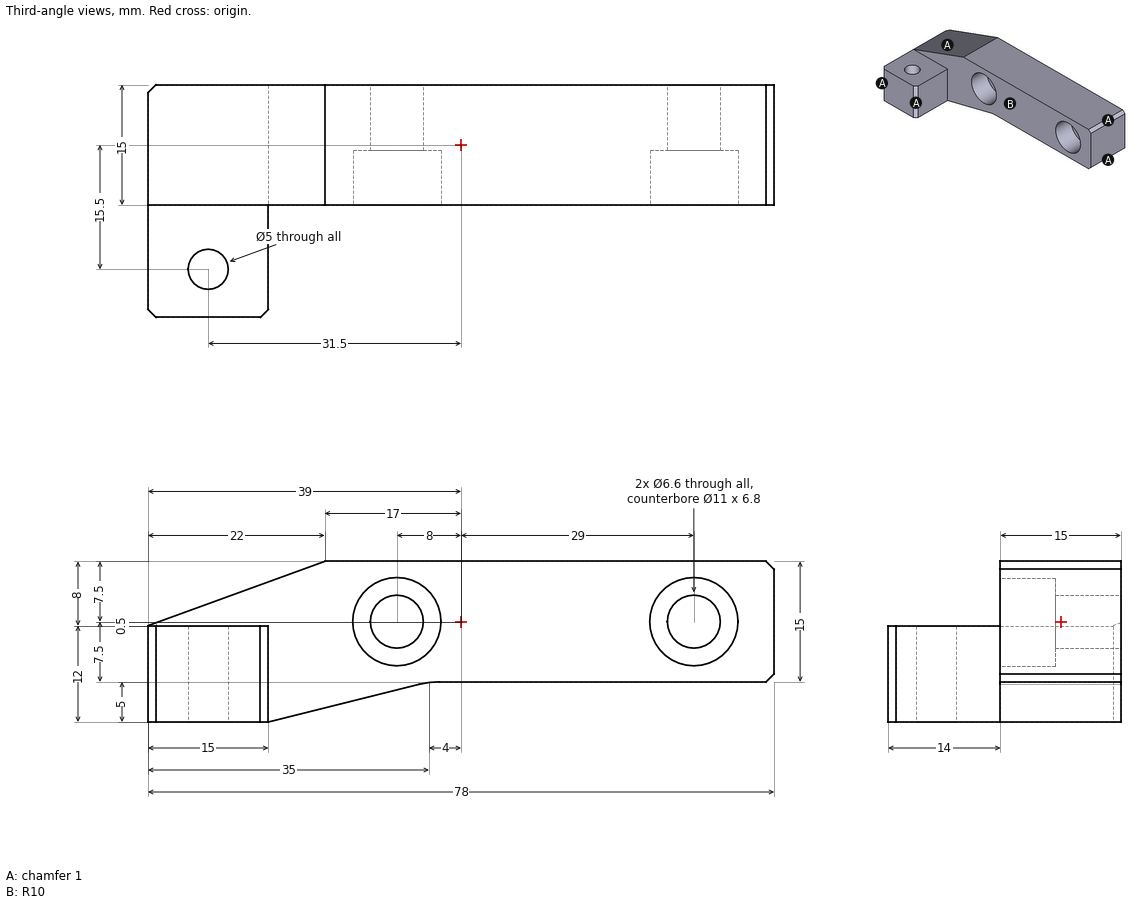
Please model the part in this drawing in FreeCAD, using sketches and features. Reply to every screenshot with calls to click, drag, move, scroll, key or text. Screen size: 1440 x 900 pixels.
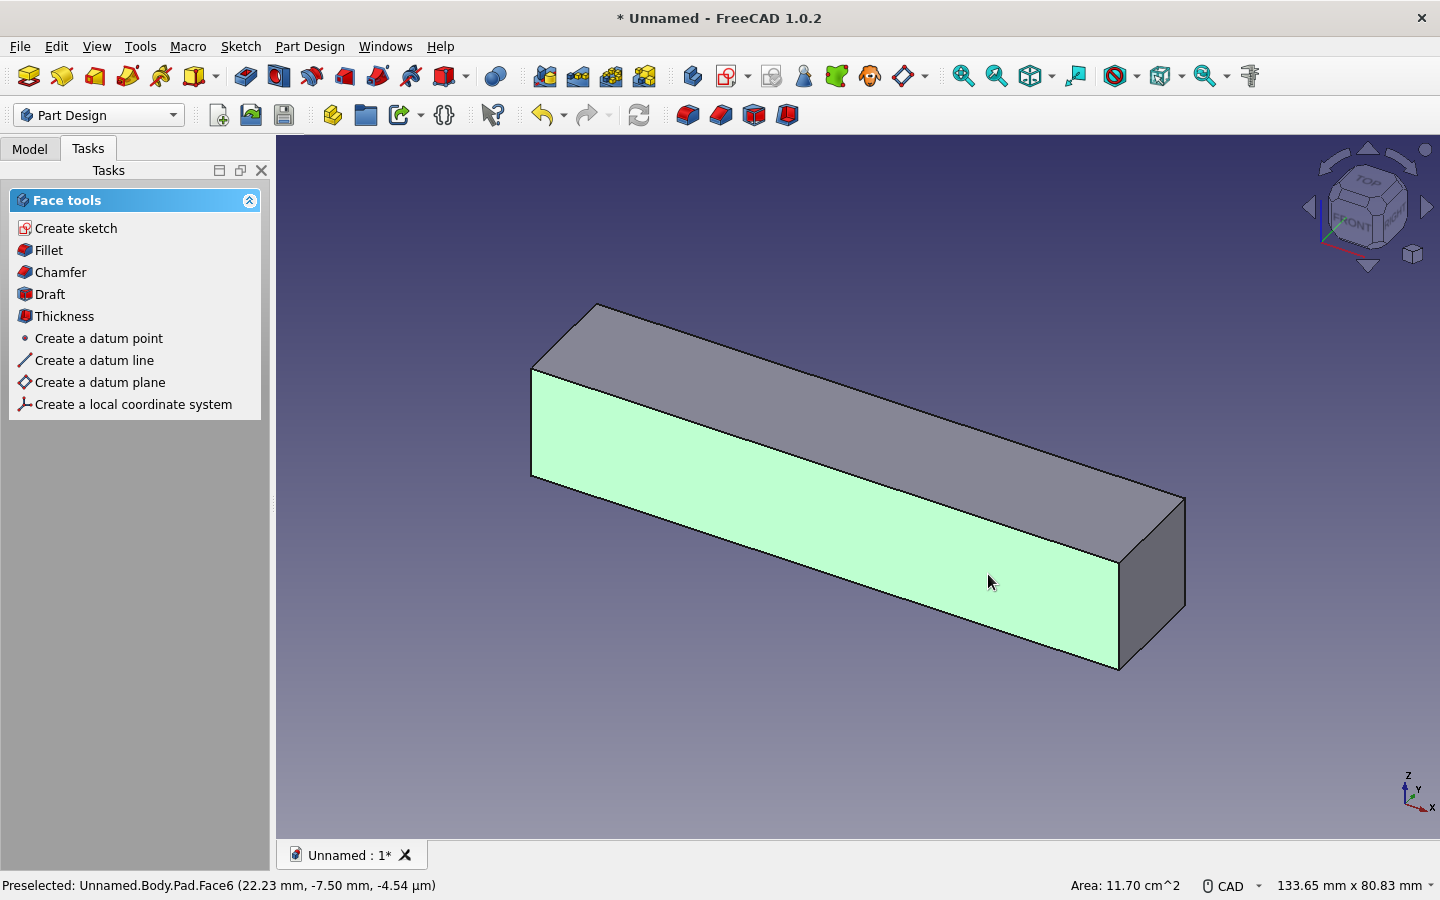
click(726, 76)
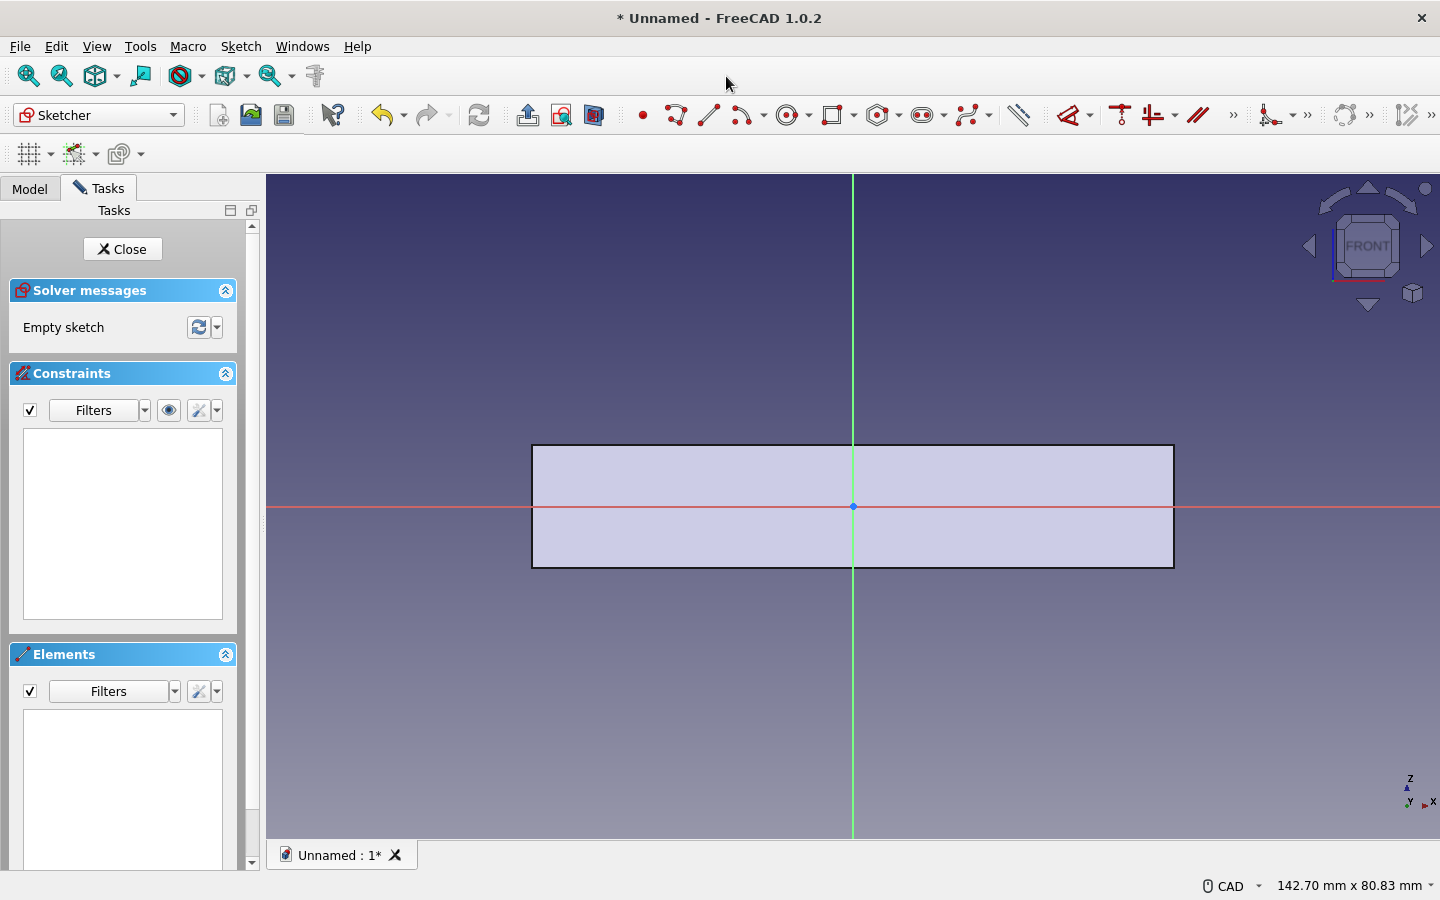
scroll(1128, 507, up, 3)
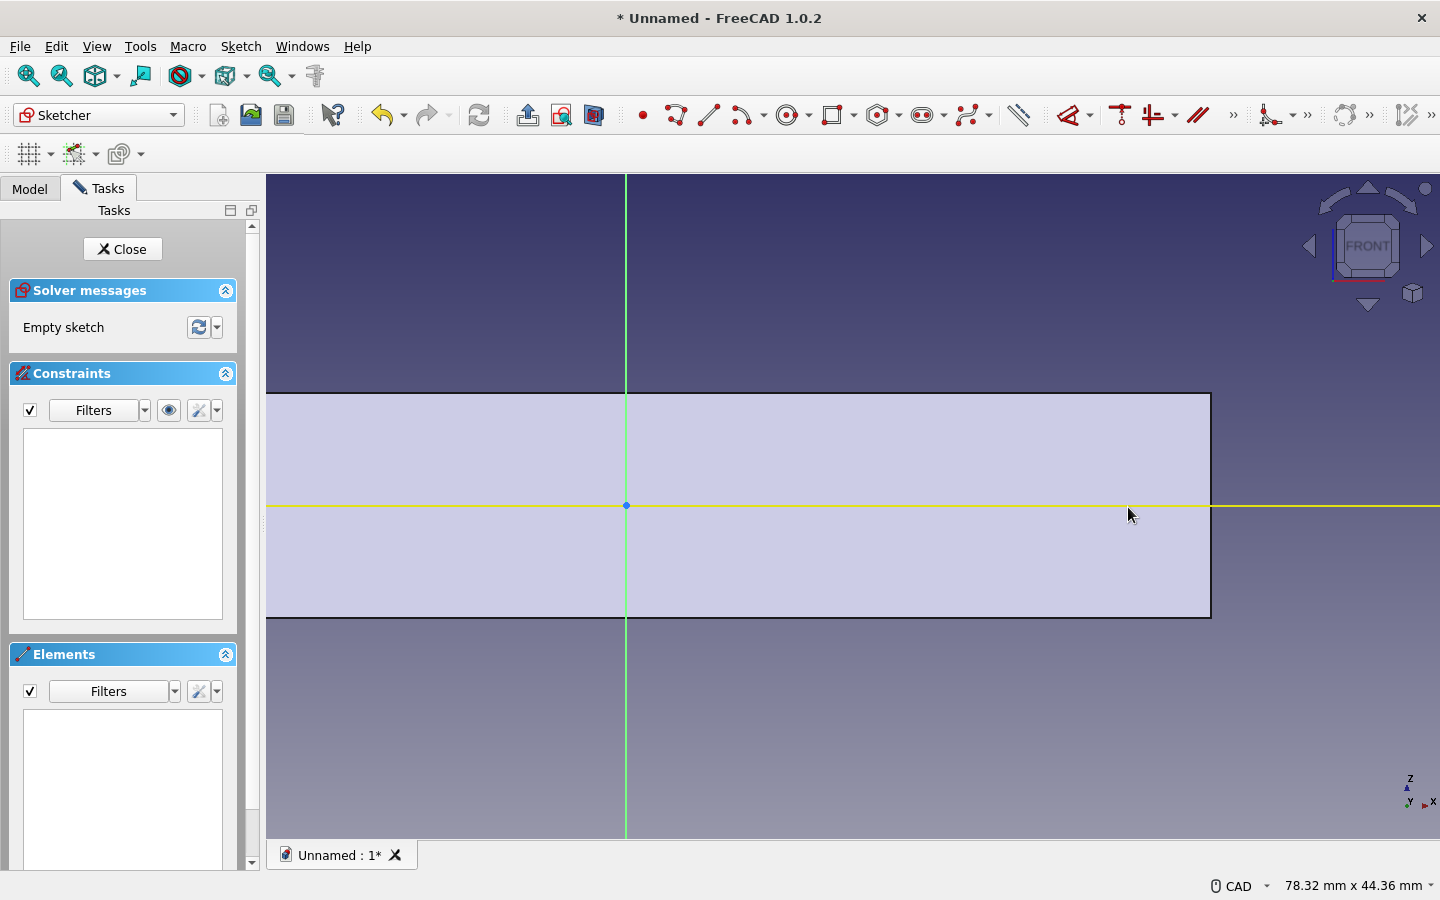
click(786, 116)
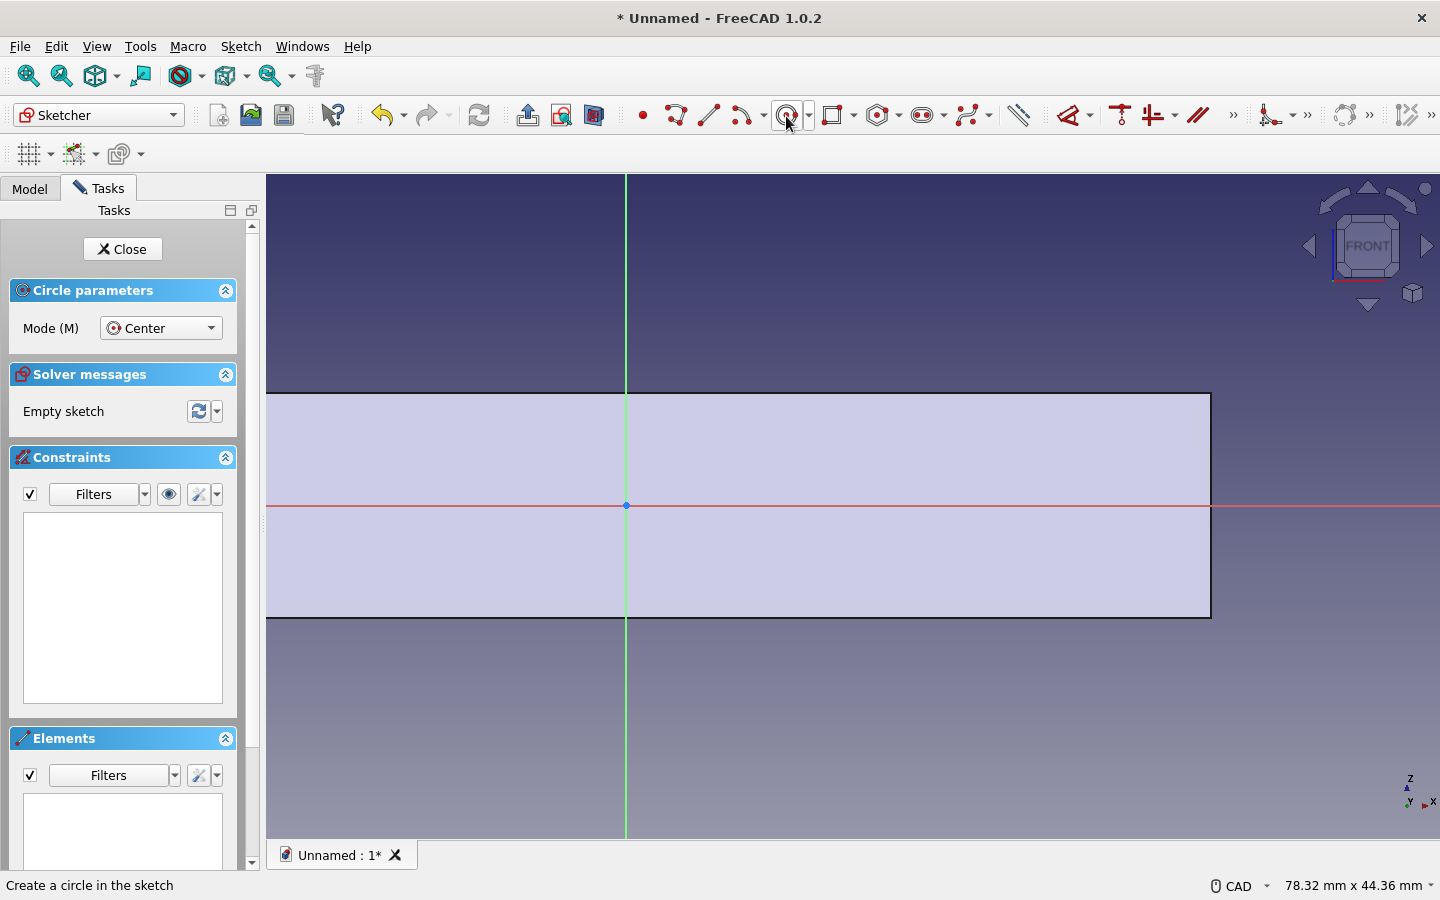
click(1061, 506)
move(1096, 471)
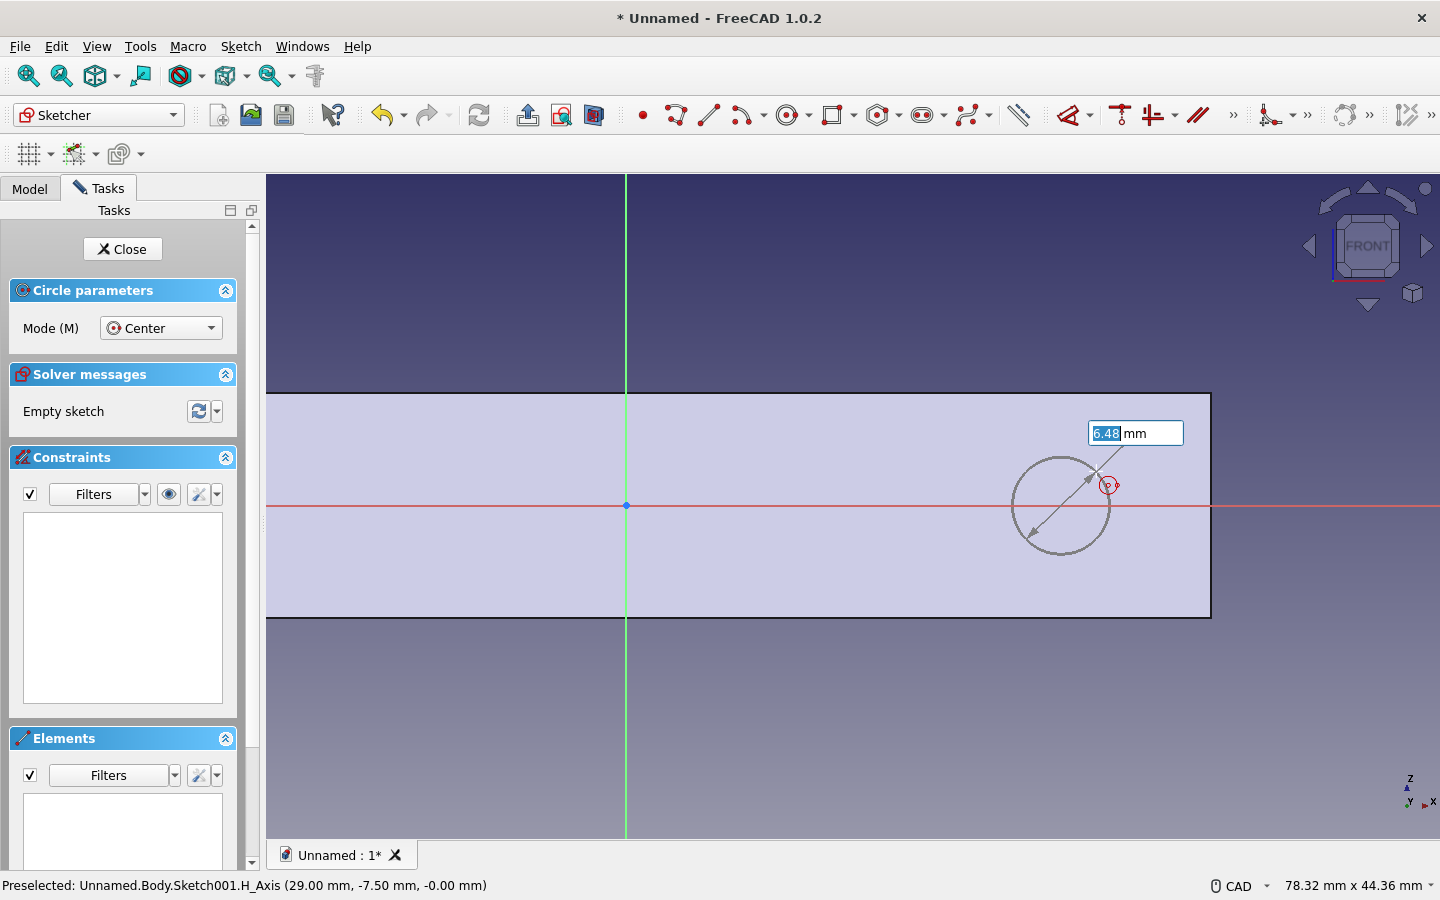
text(6.6)
key(Return)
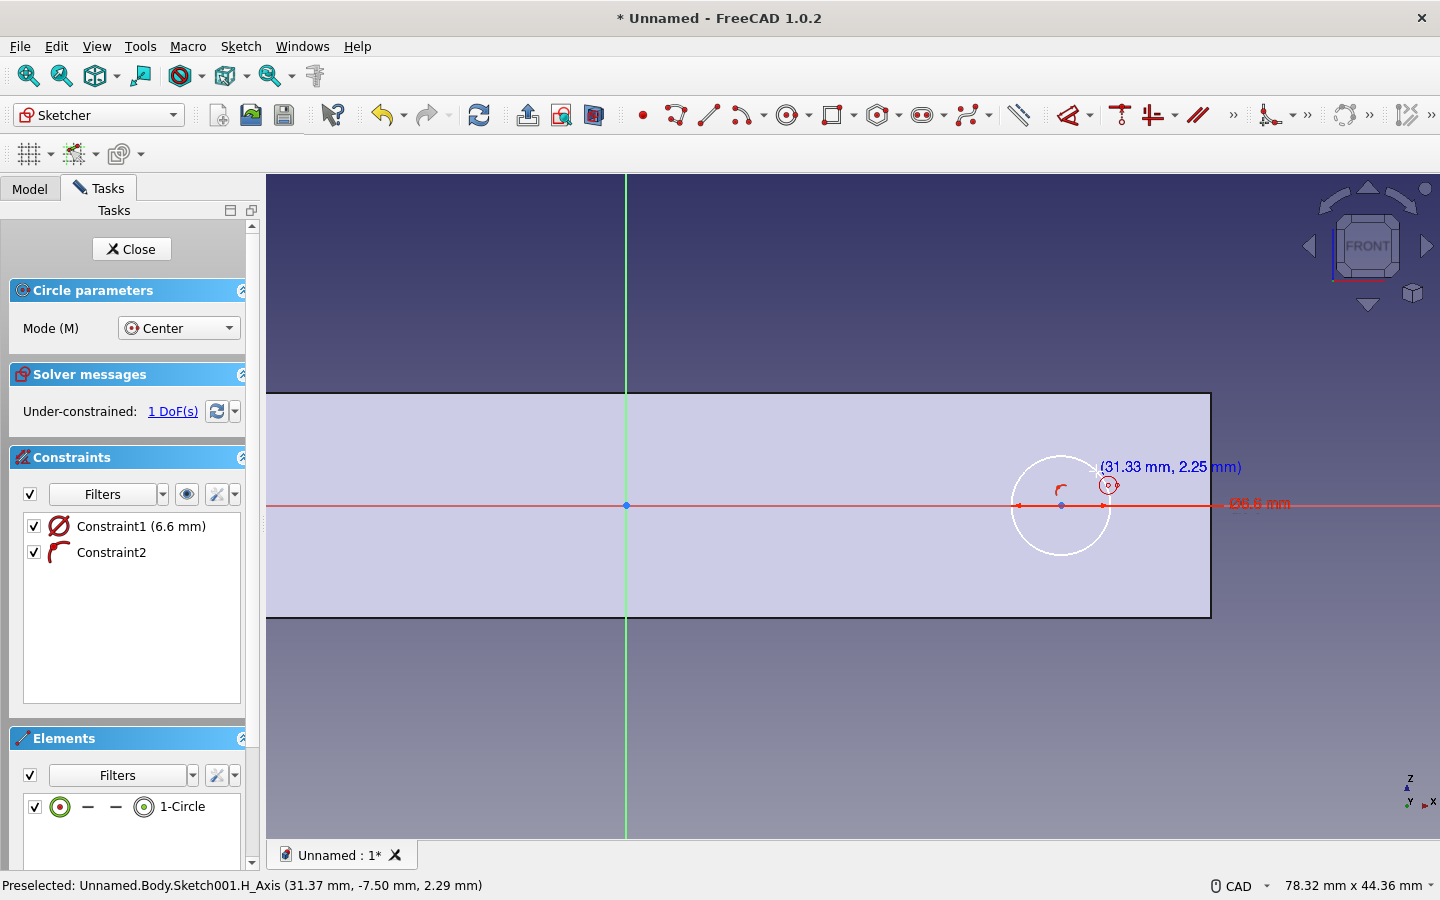
click(506, 506)
move(541, 471)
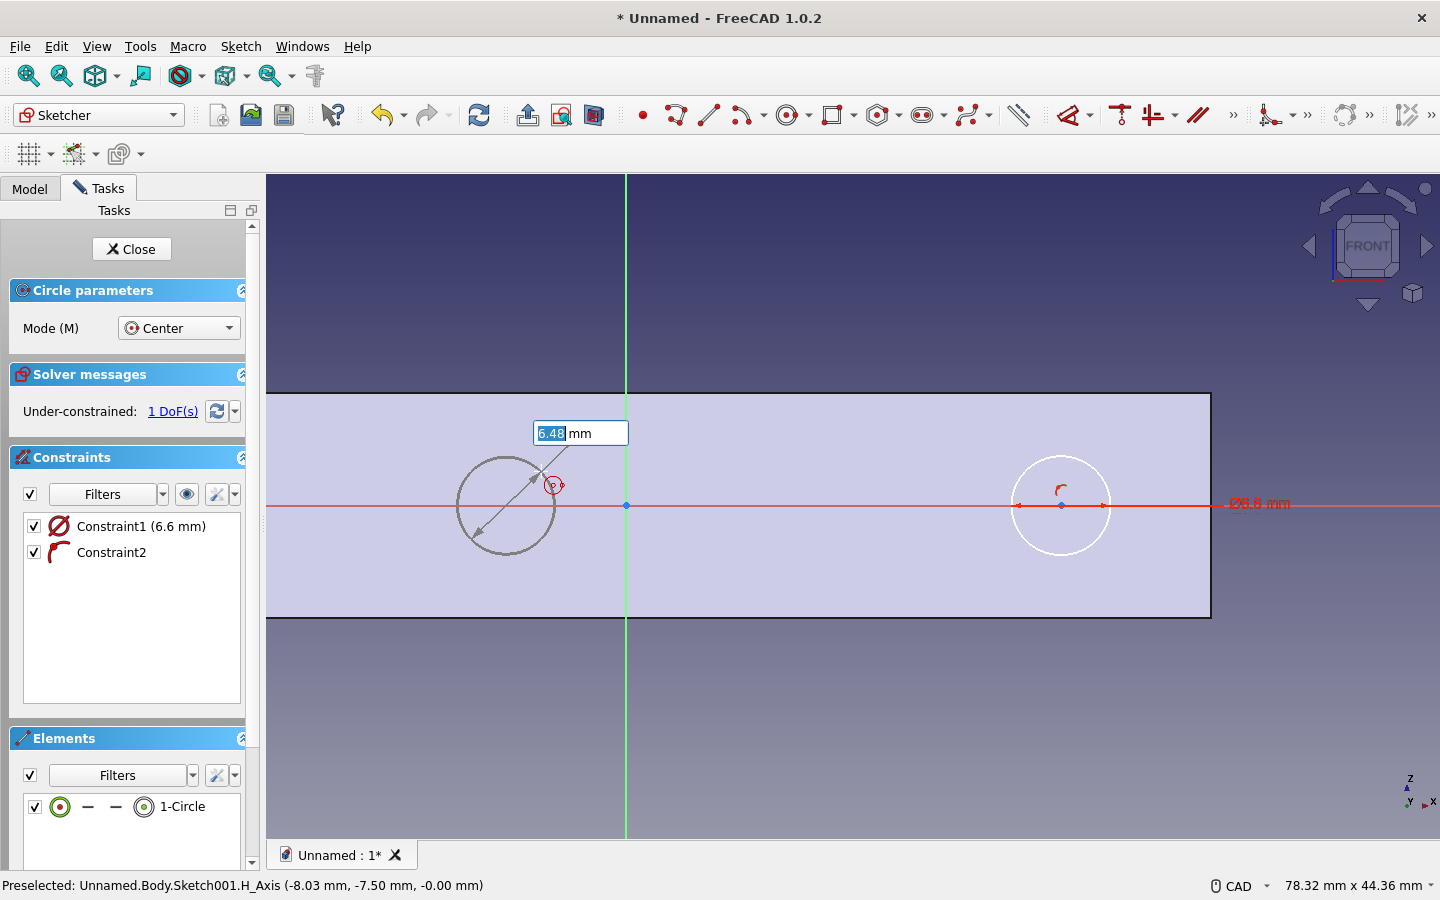
text(6.6)
key(Return)
key(Escape)